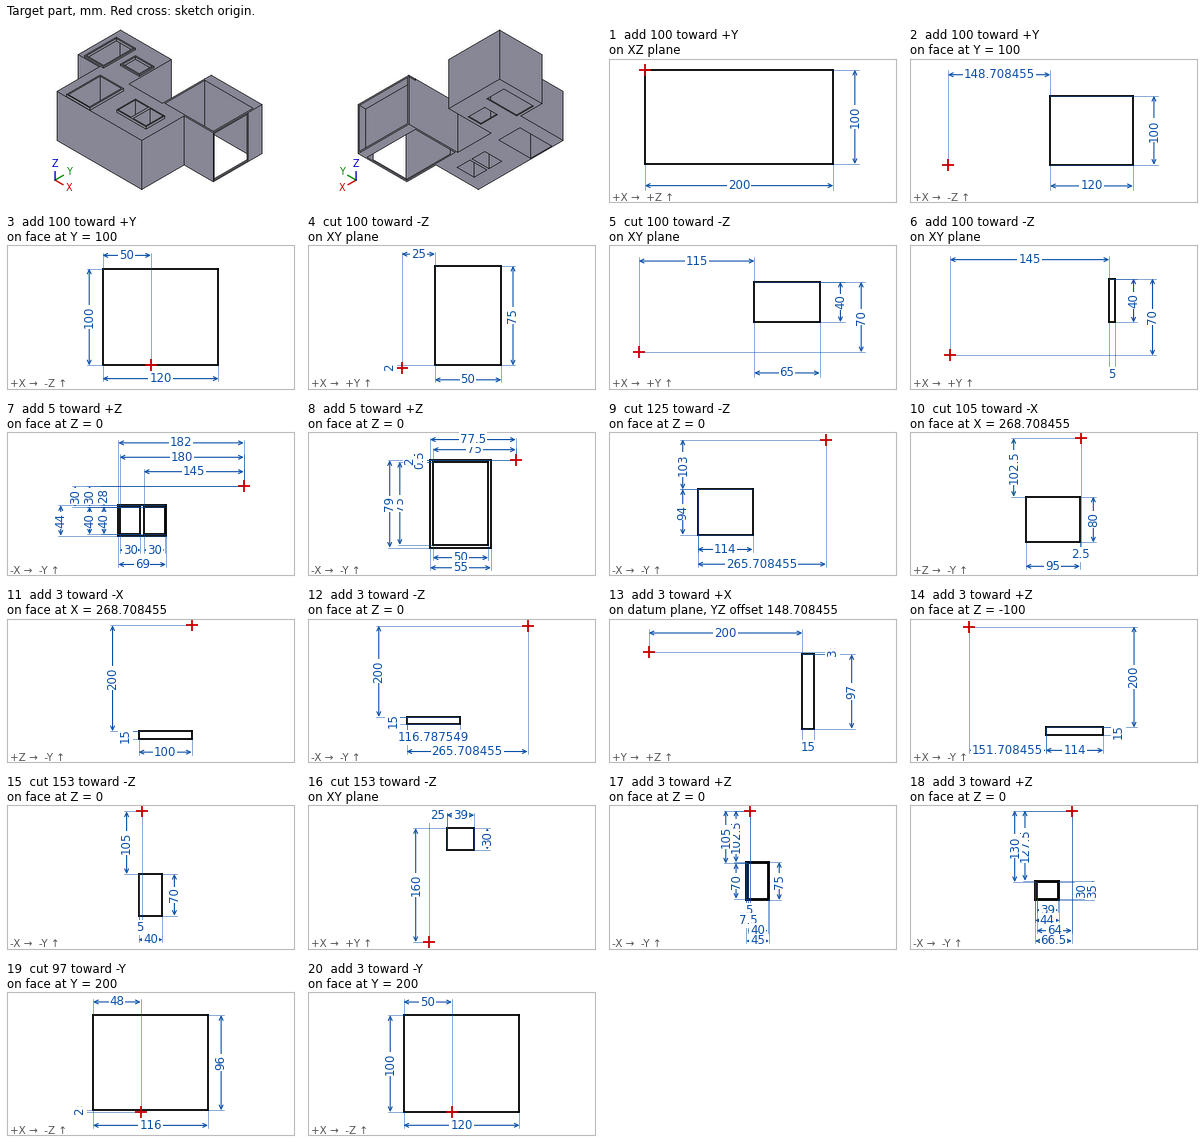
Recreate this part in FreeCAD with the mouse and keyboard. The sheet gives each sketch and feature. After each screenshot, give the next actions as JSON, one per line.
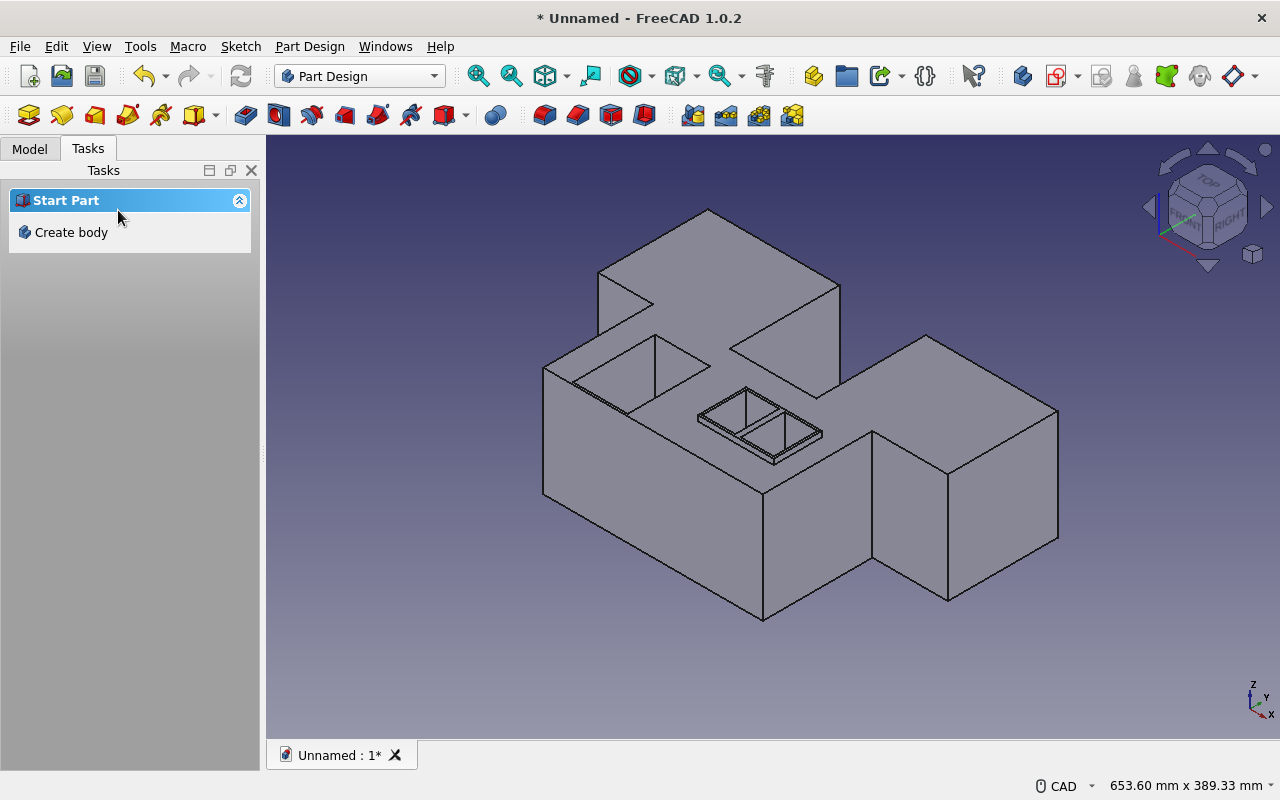
{"action": "left_click", "coordinate": [936, 394]}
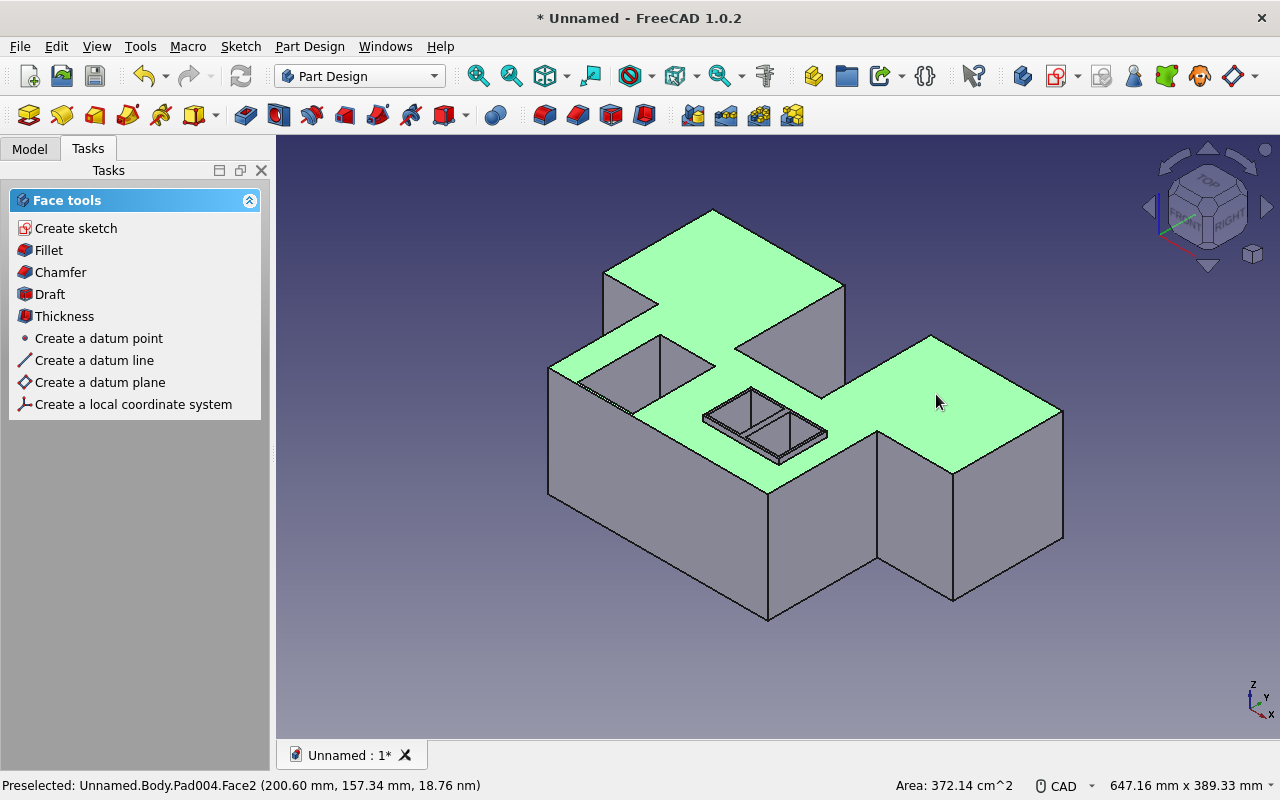
{"action": "left_click", "coordinate": [1056, 76]}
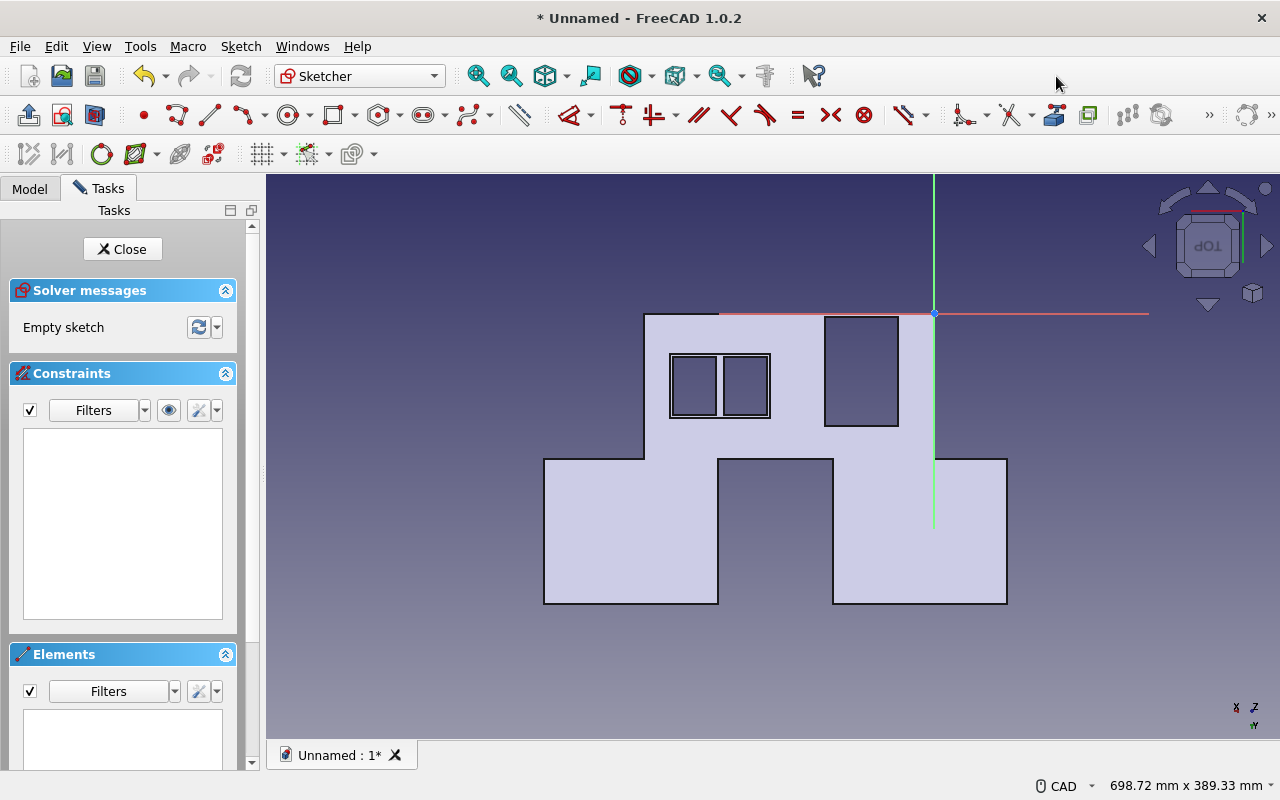
{"action": "scroll", "coordinate": [953, 335], "scroll_direction": "up", "scroll_amount": 6}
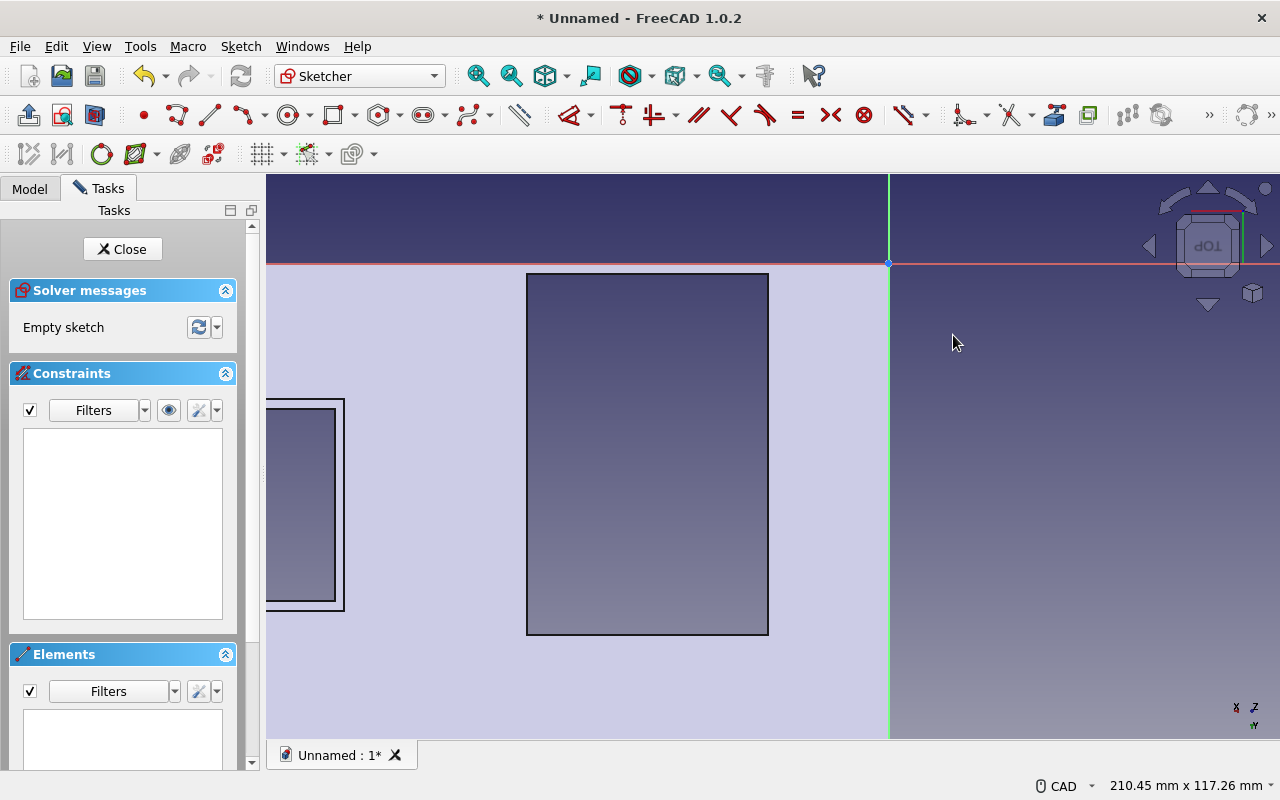
{"action": "left_click", "coordinate": [332, 116]}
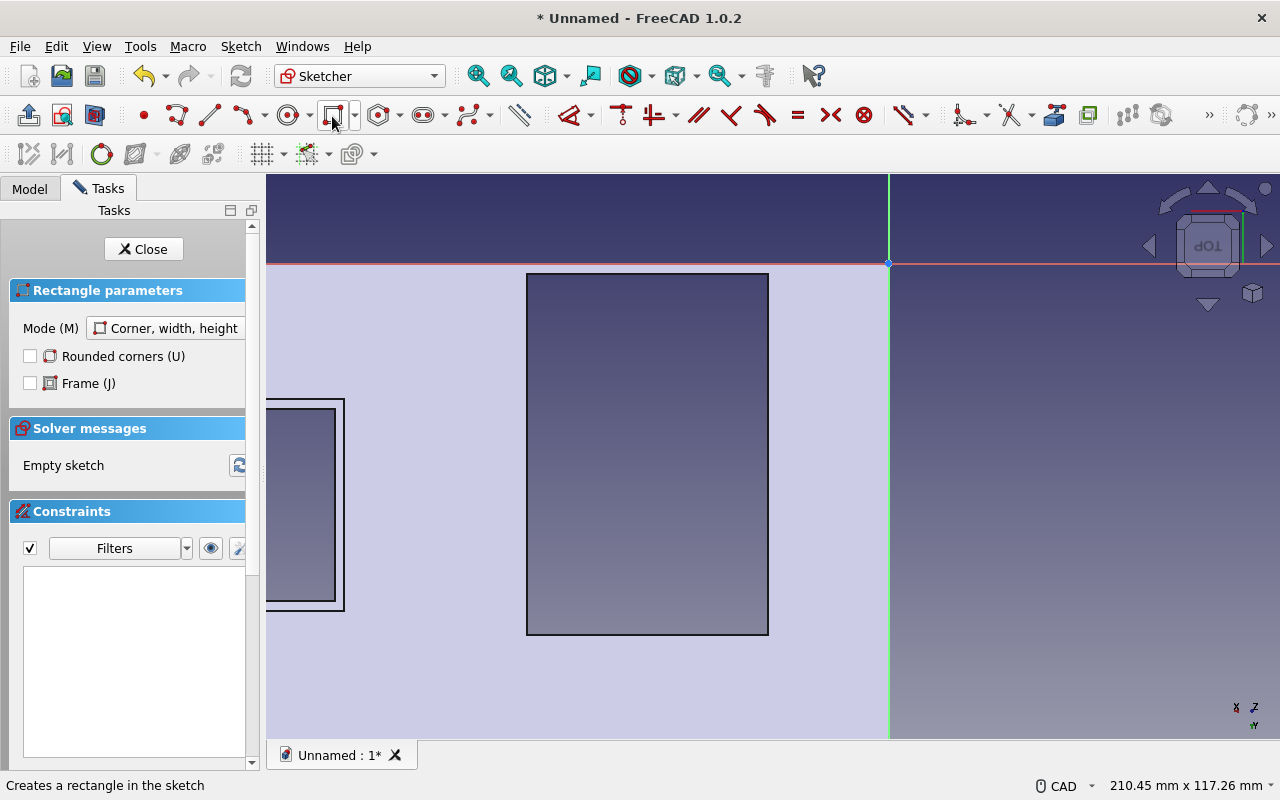
{"action": "scroll", "coordinate": [515, 266], "scroll_direction": "up", "scroll_amount": 10}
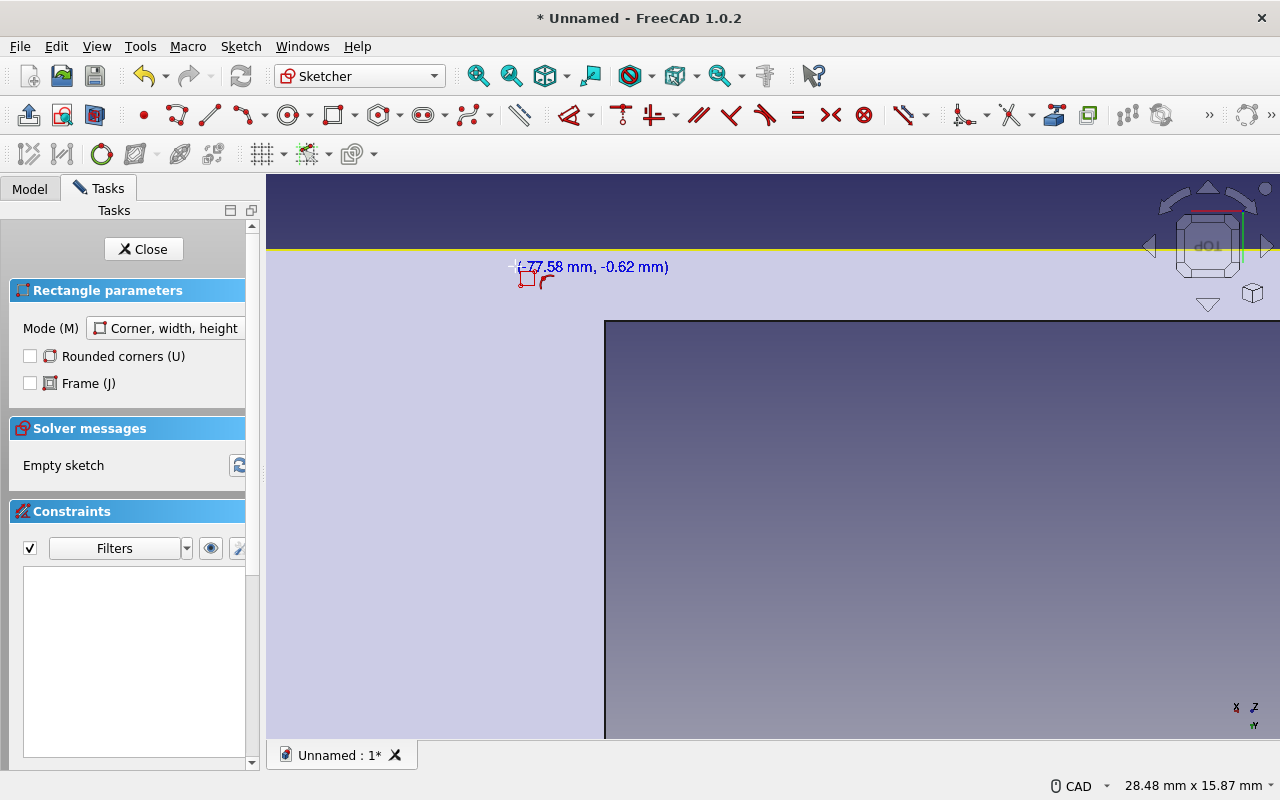
{"action": "left_click", "coordinate": [516, 268]}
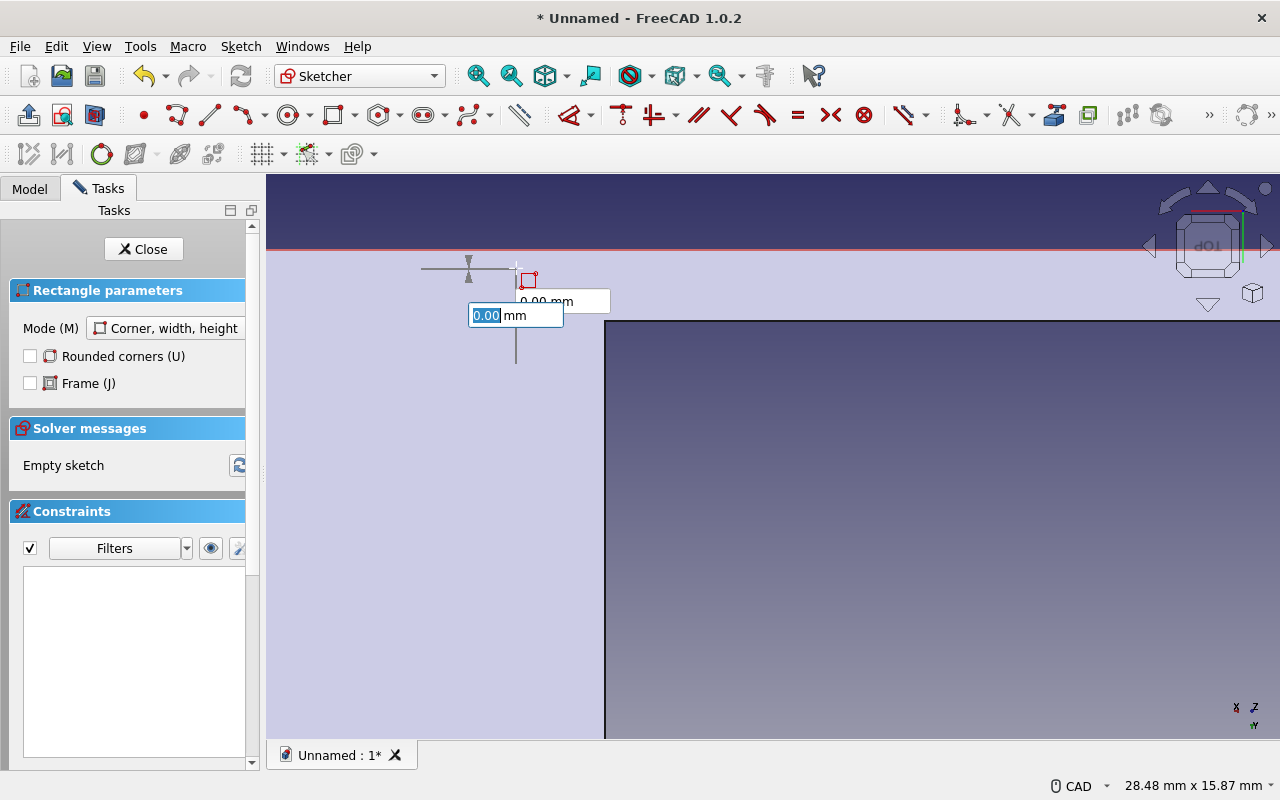
{"action": "scroll", "coordinate": [518, 267], "scroll_direction": "down", "scroll_amount": 10}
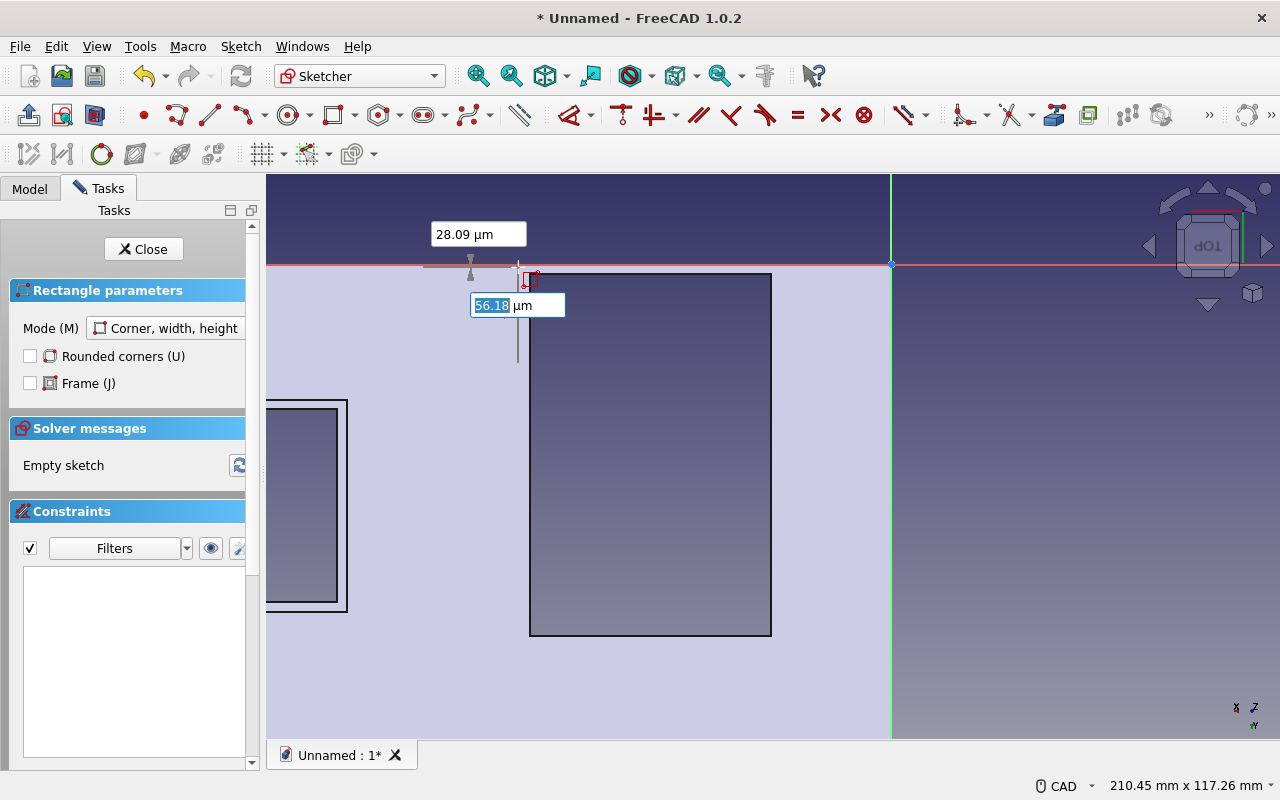
{"action": "left_click", "coordinate": [783, 648]}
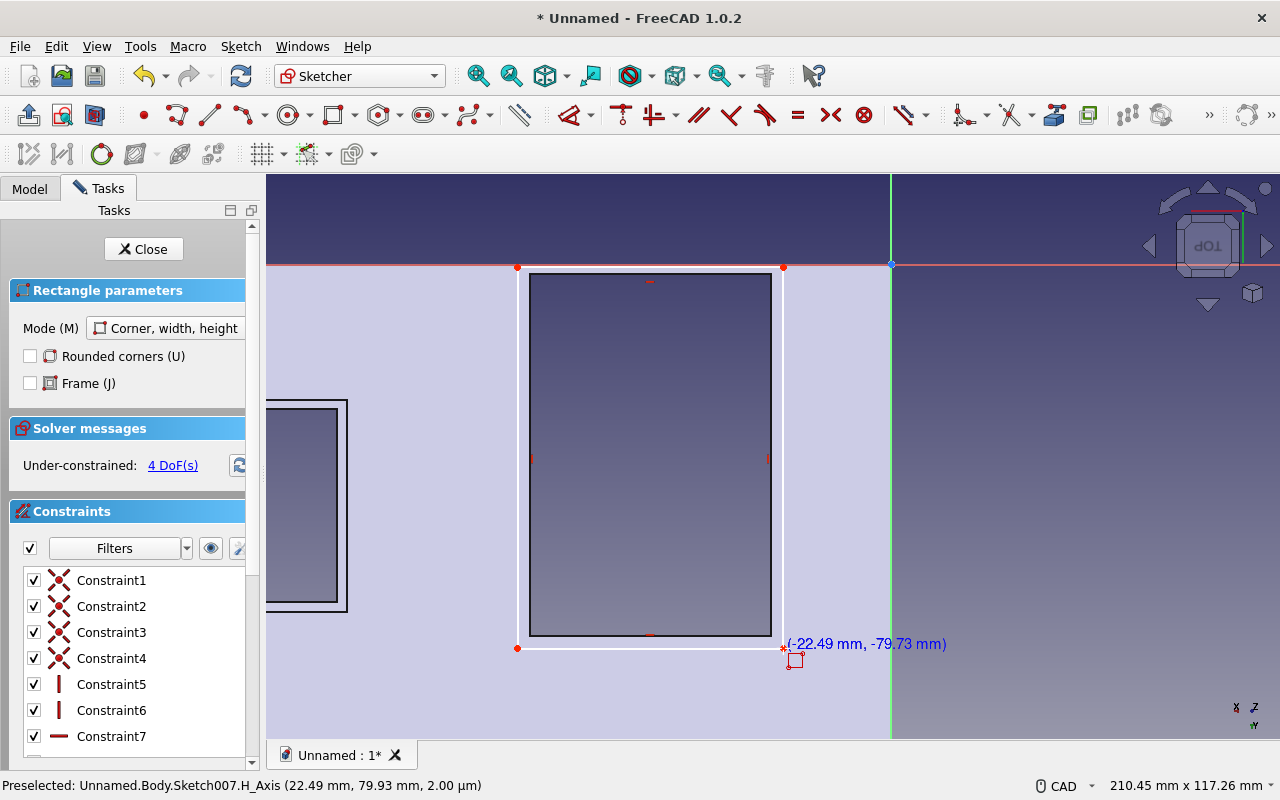
{"action": "scroll", "coordinate": [530, 274], "scroll_direction": "up", "scroll_amount": 4}